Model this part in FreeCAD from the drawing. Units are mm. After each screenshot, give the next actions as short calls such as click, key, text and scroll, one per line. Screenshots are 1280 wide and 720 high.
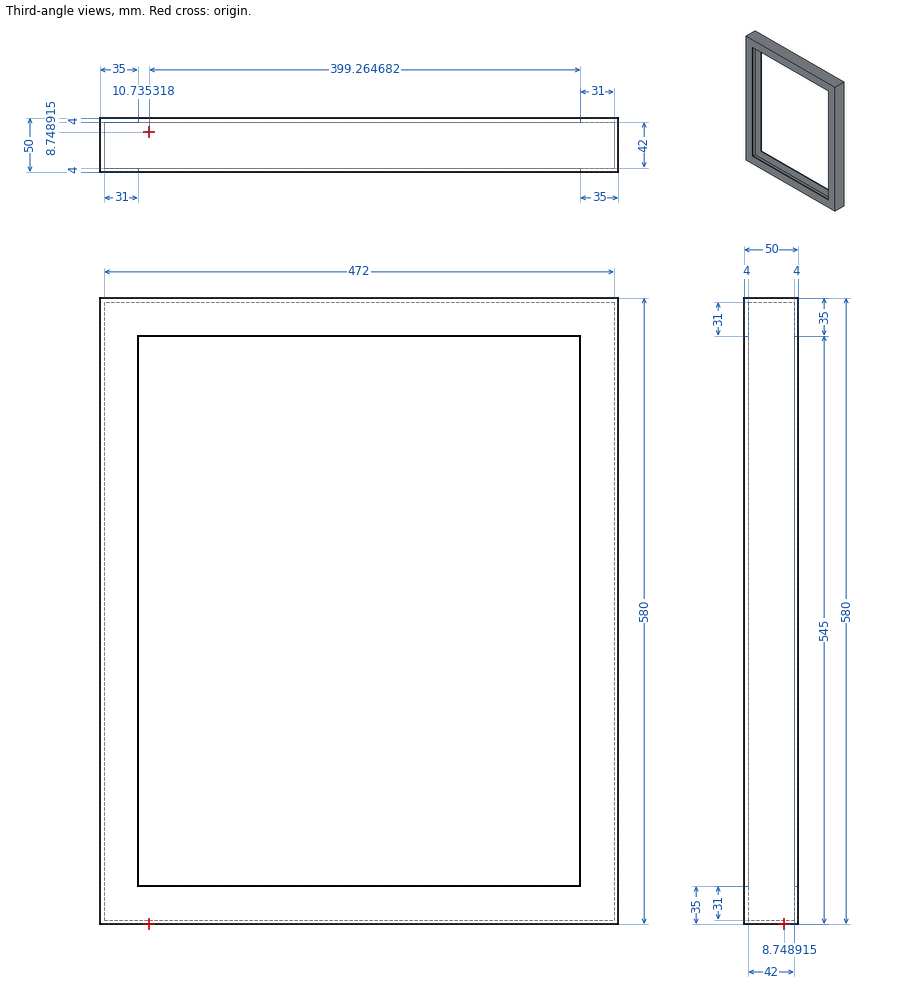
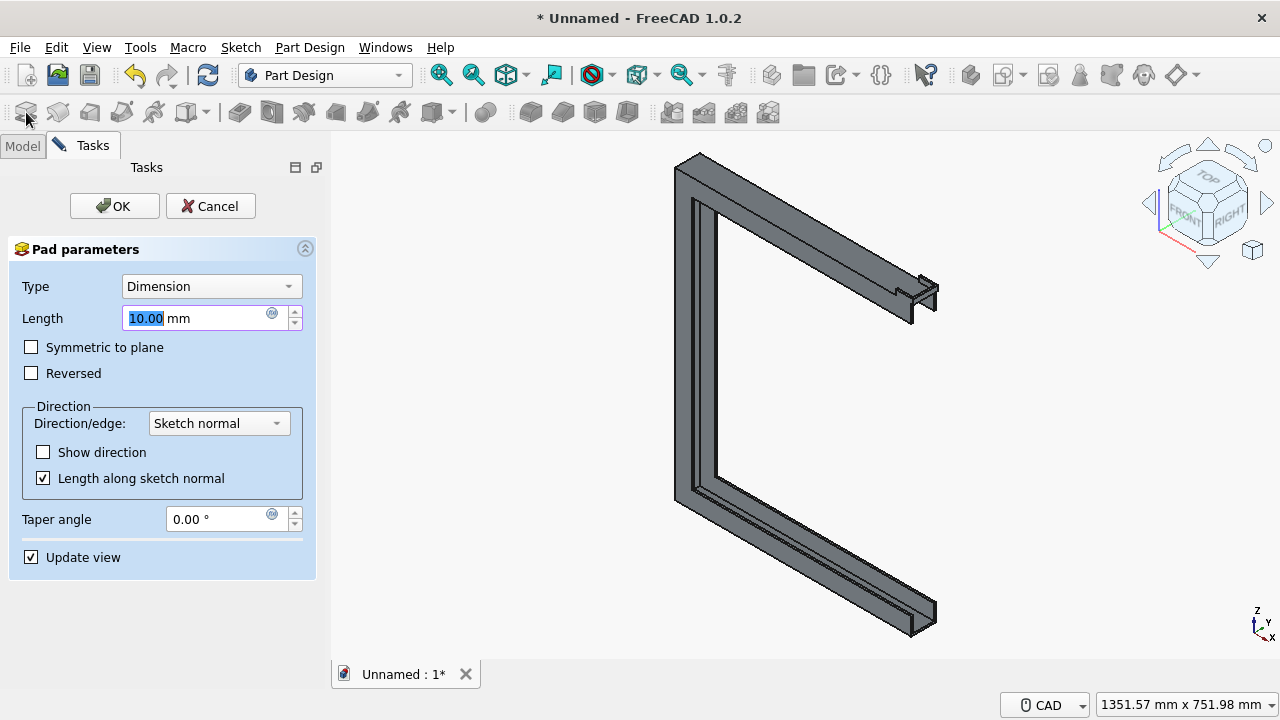
text(580)
key(Tab)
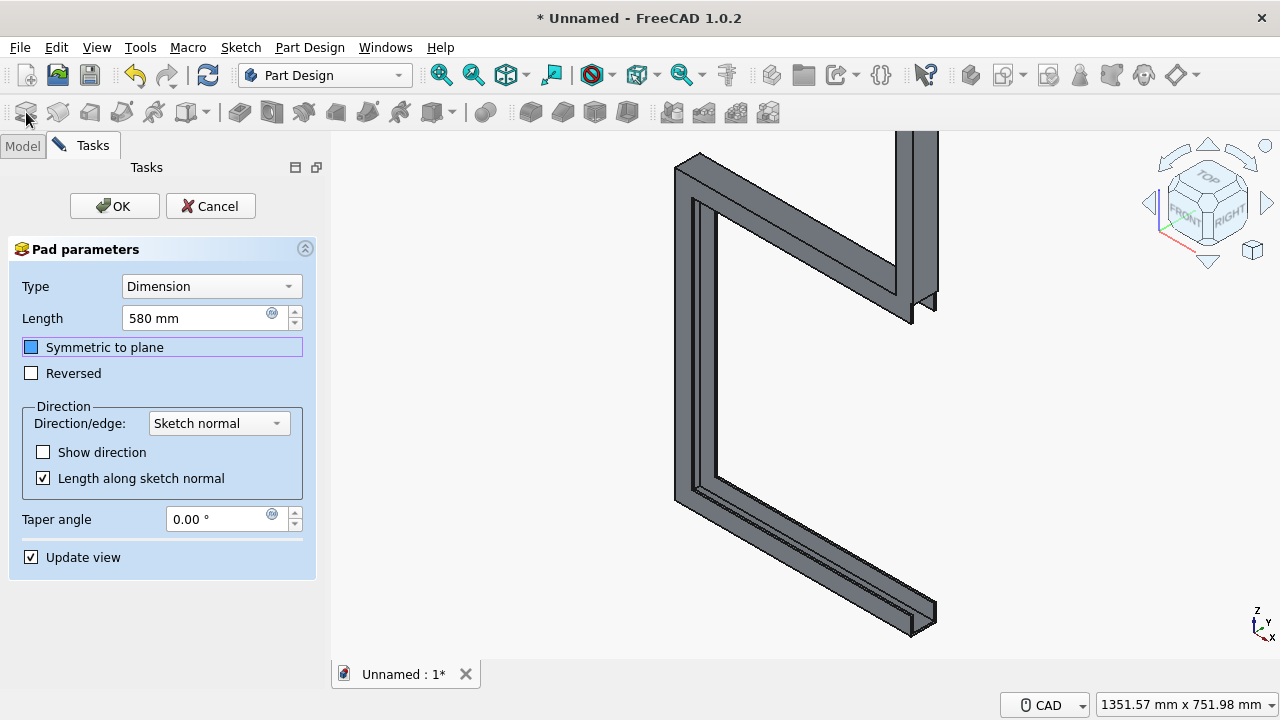
click(30, 373)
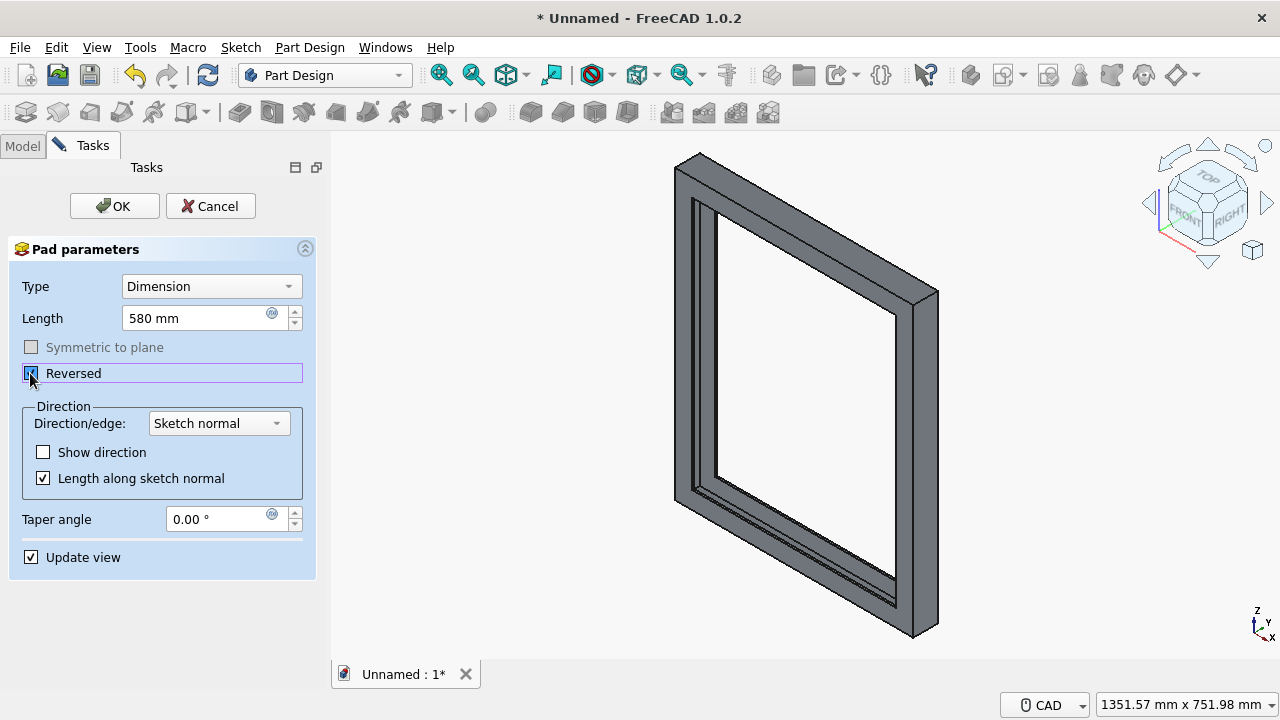
click(115, 206)